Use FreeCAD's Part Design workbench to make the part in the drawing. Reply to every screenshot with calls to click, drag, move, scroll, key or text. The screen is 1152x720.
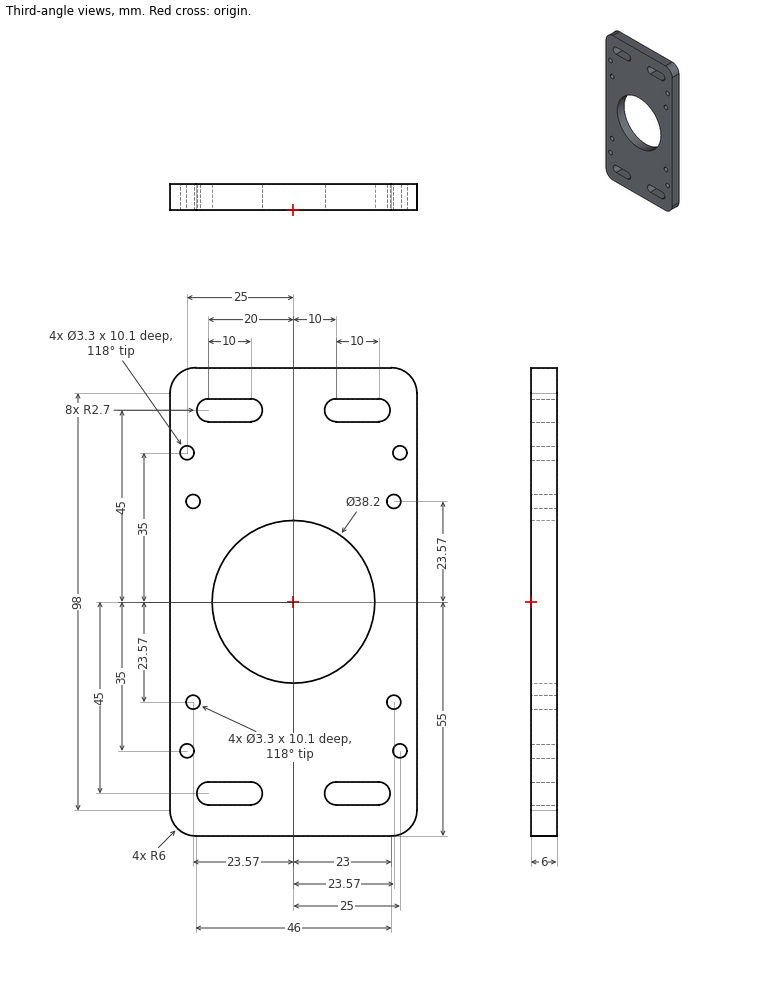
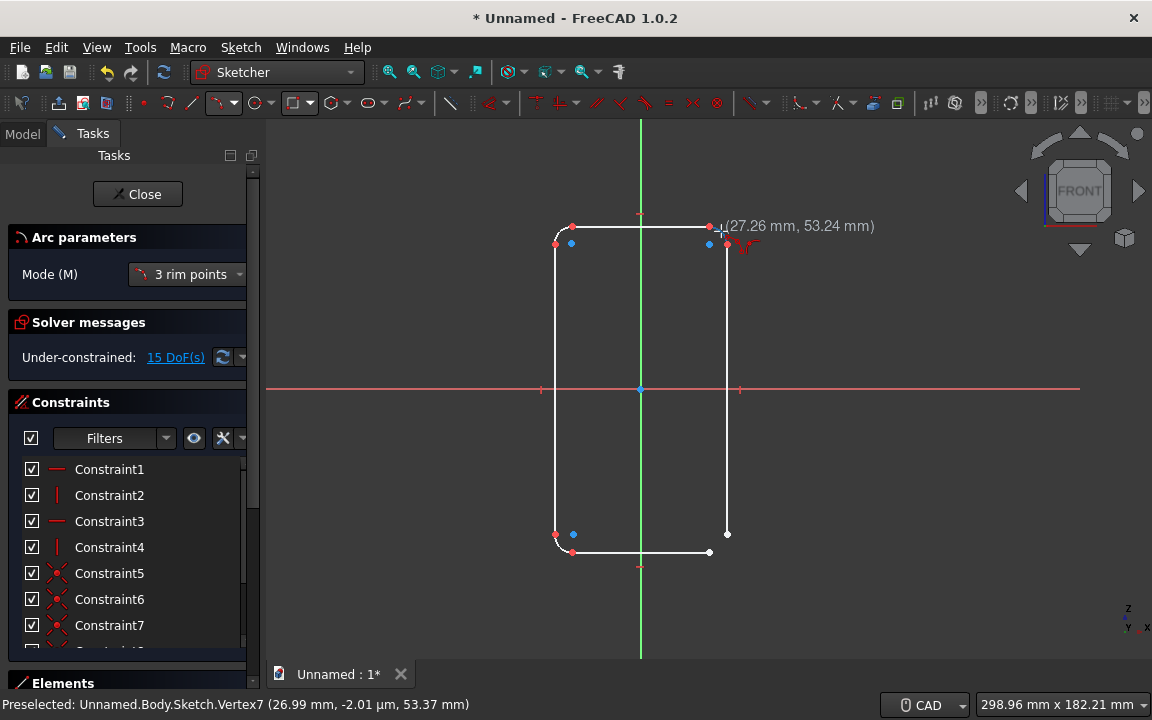
click(727, 535)
click(709, 553)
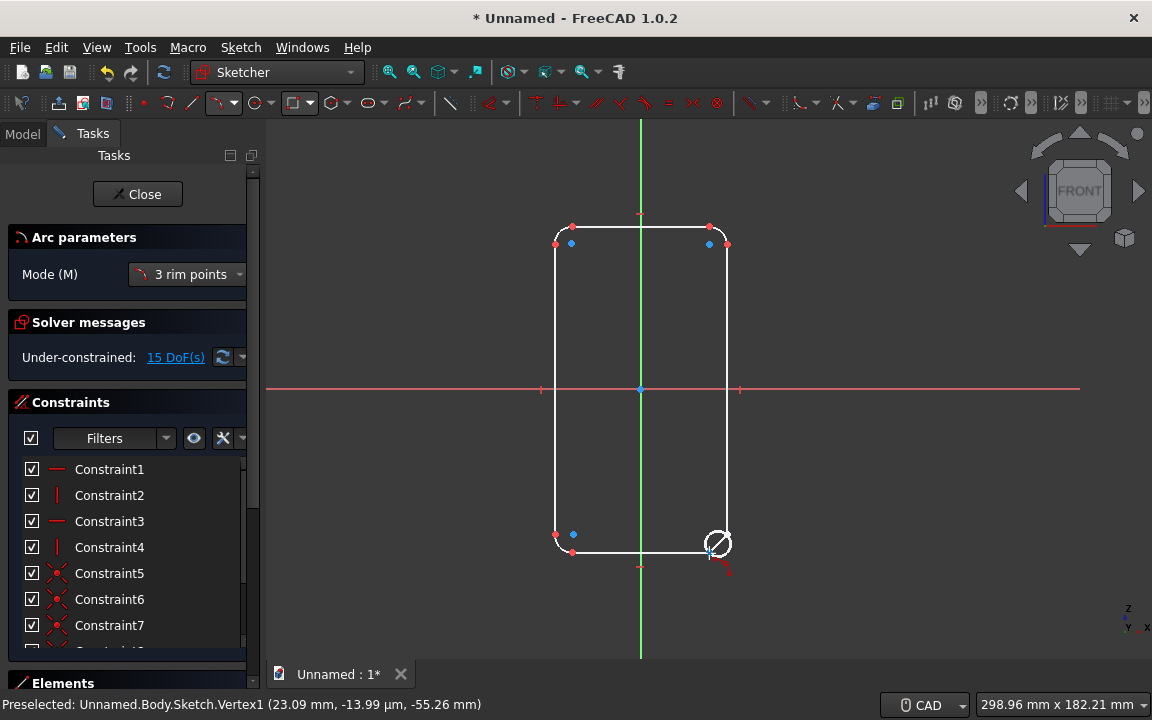
scroll(721, 547, up, 6)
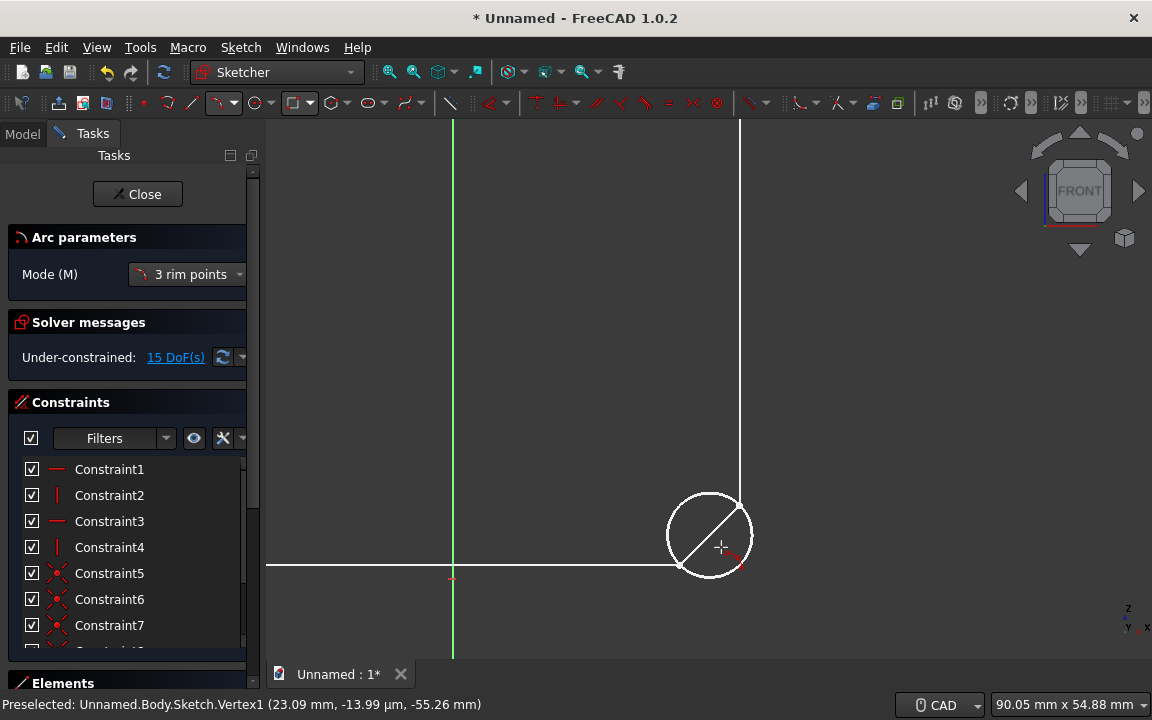
click(721, 545)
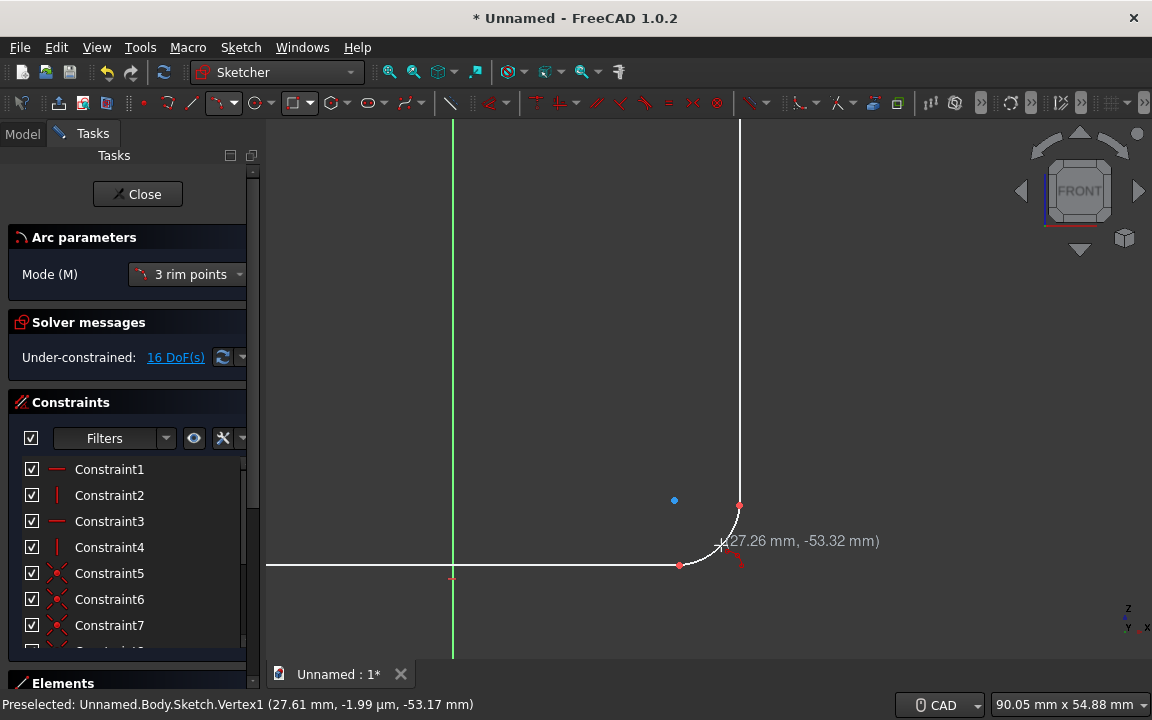
click(256, 104)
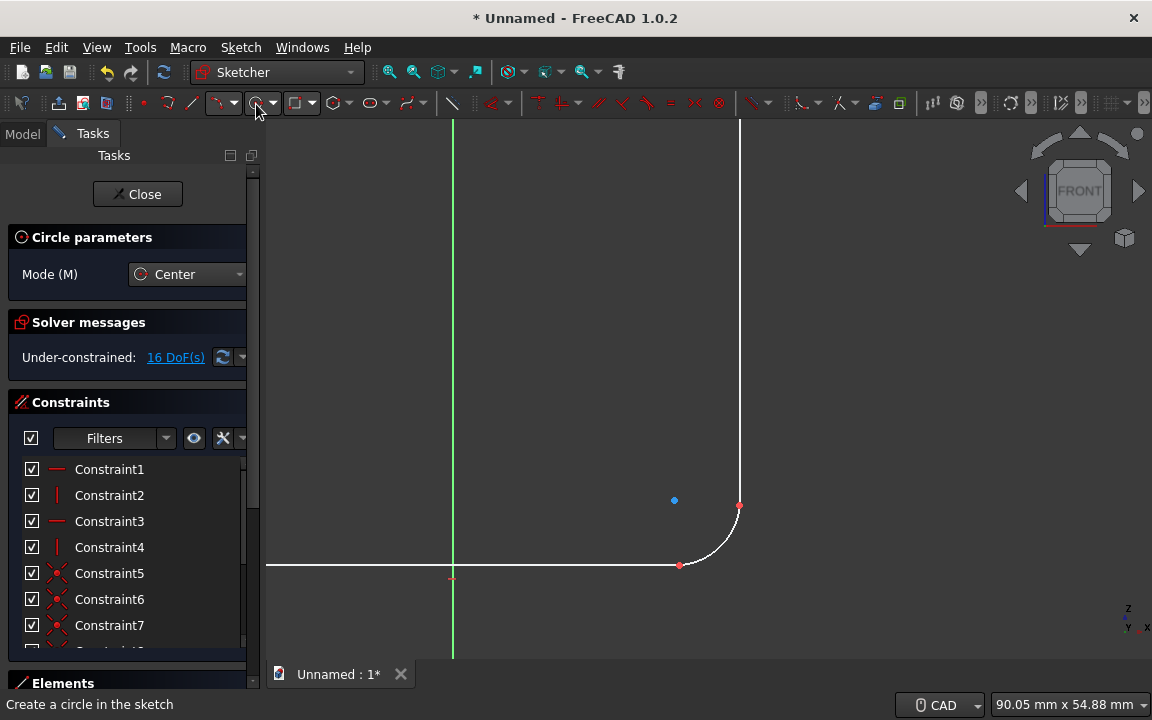
scroll(721, 547, down, 6)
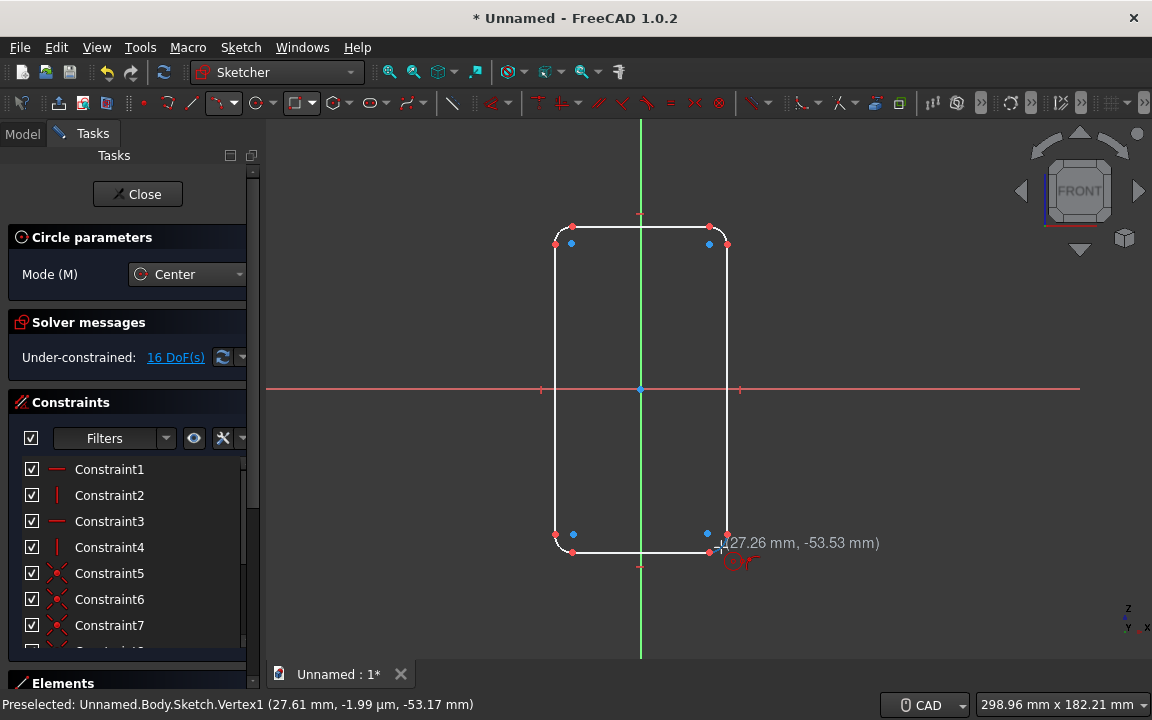
click(641, 389)
move(681, 349)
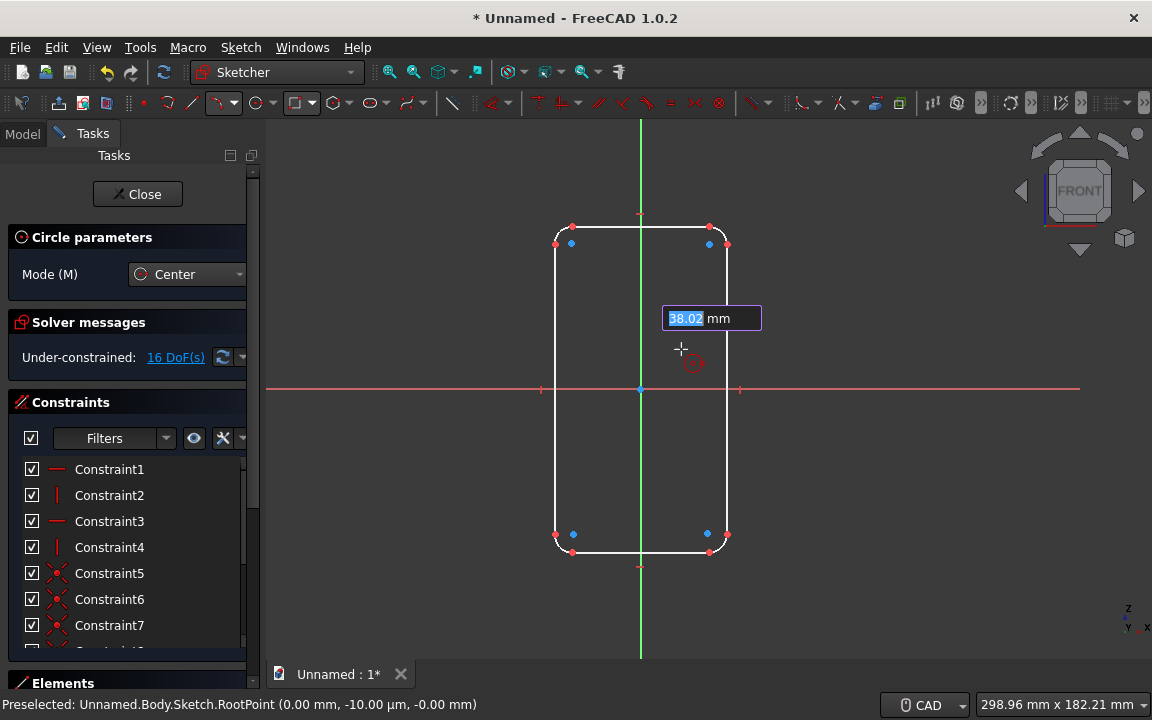
text(38.2)
key(Return)
key(Escape)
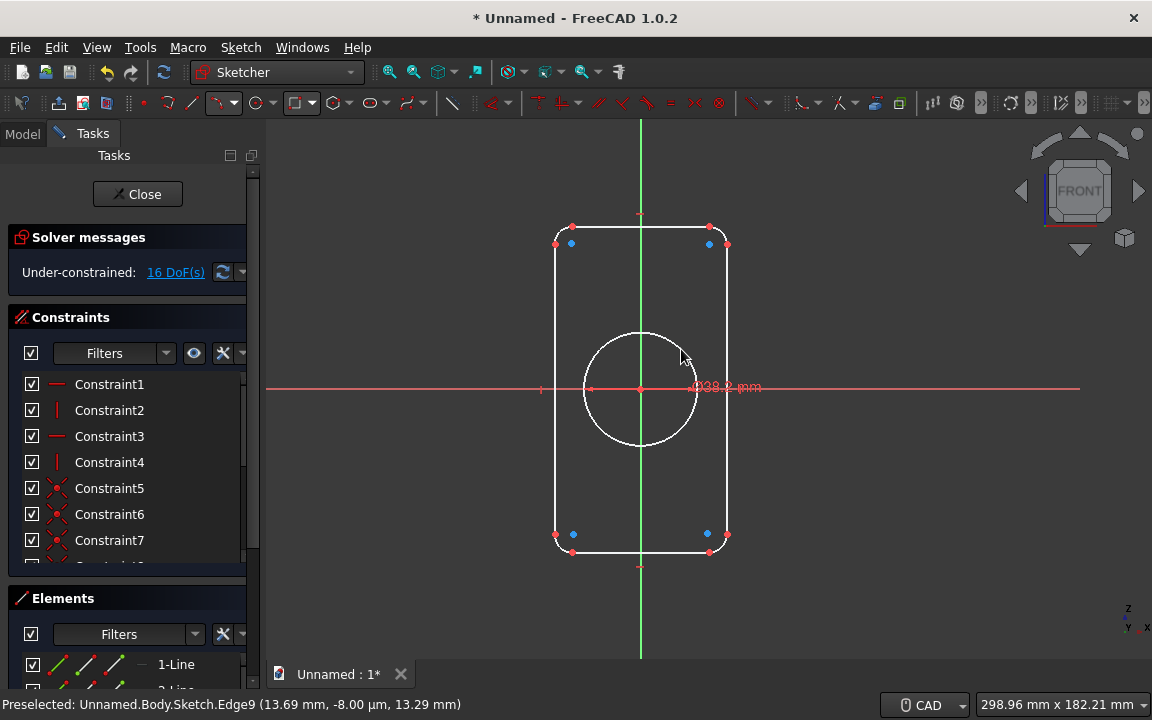
click(668, 553)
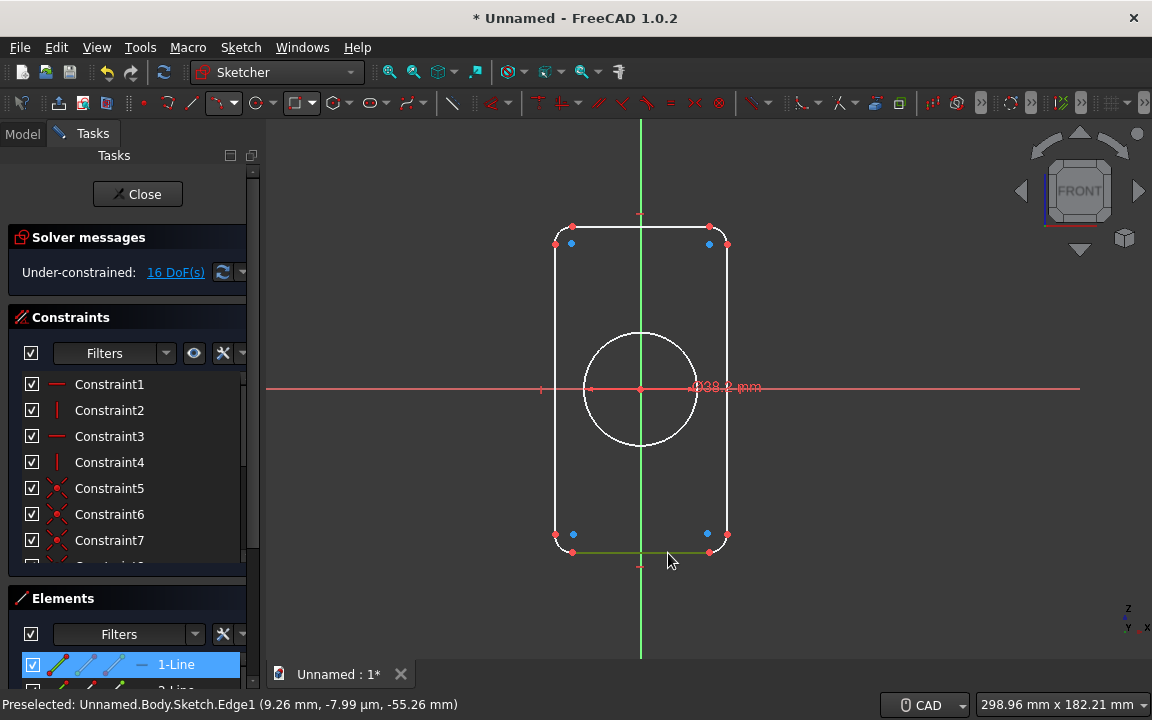
click(560, 547)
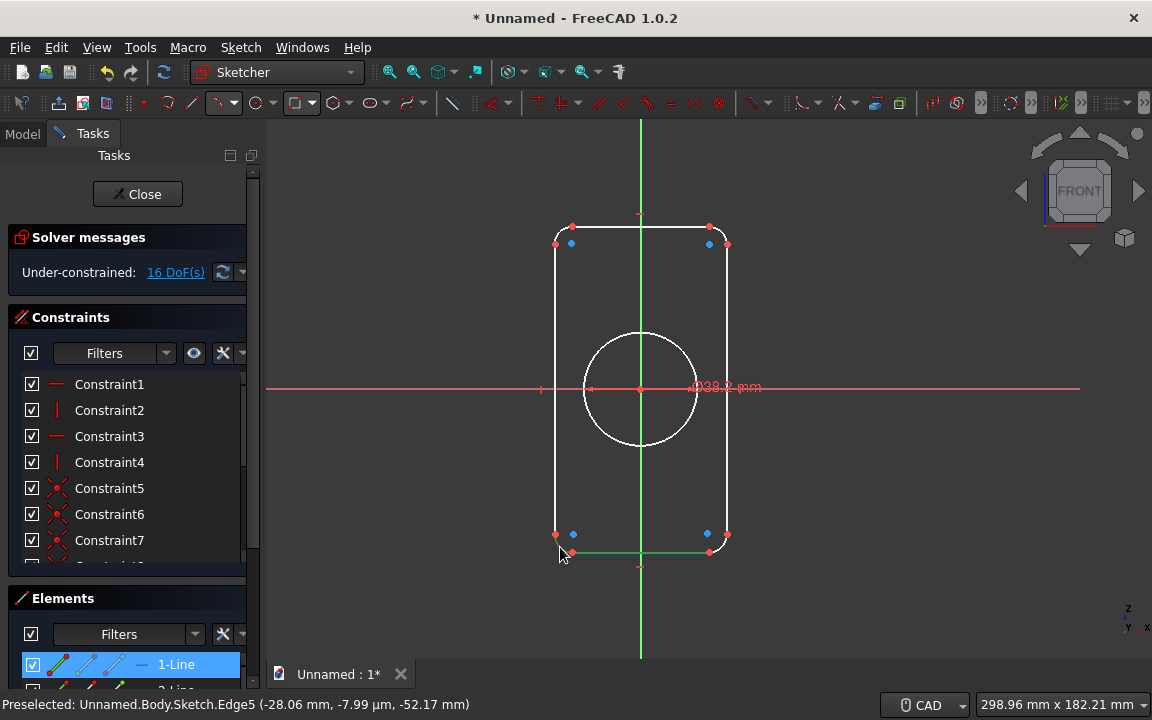
key(t)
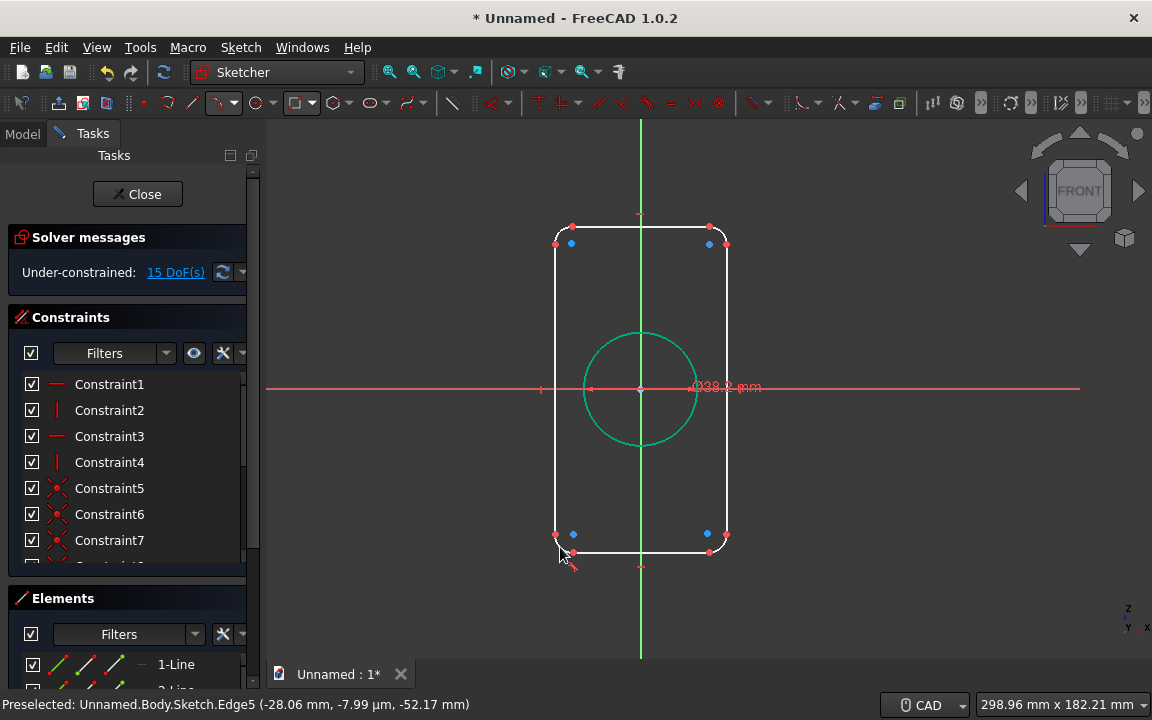
click(668, 553)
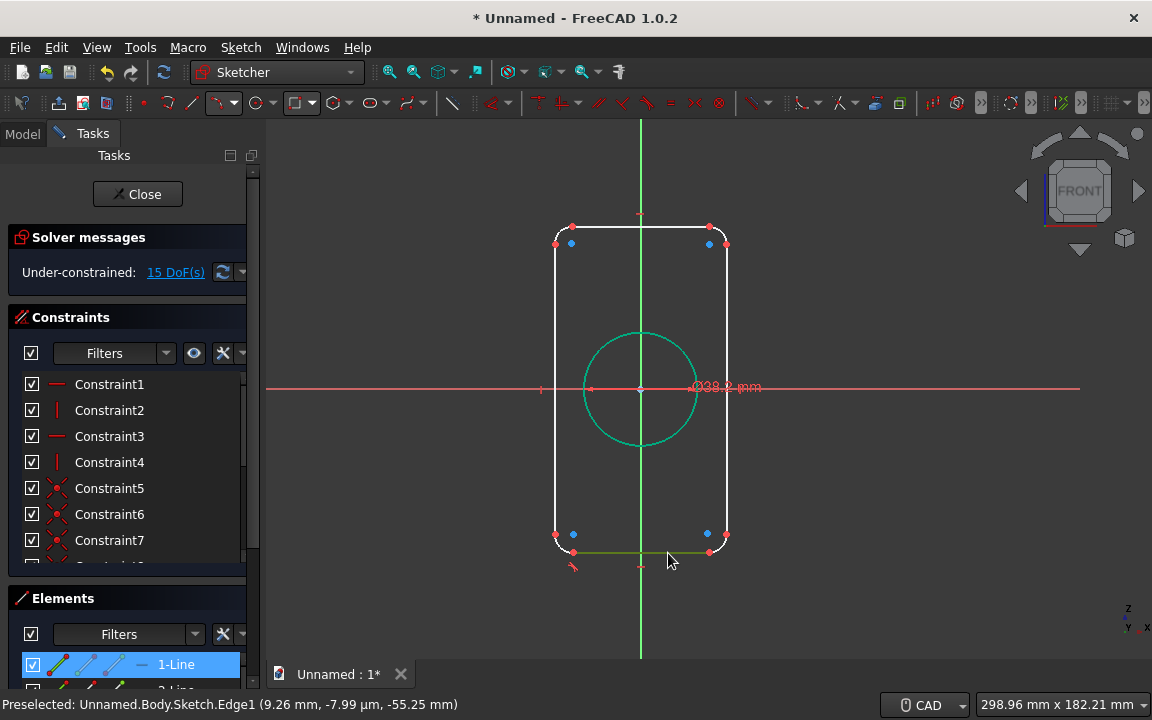
click(721, 547)